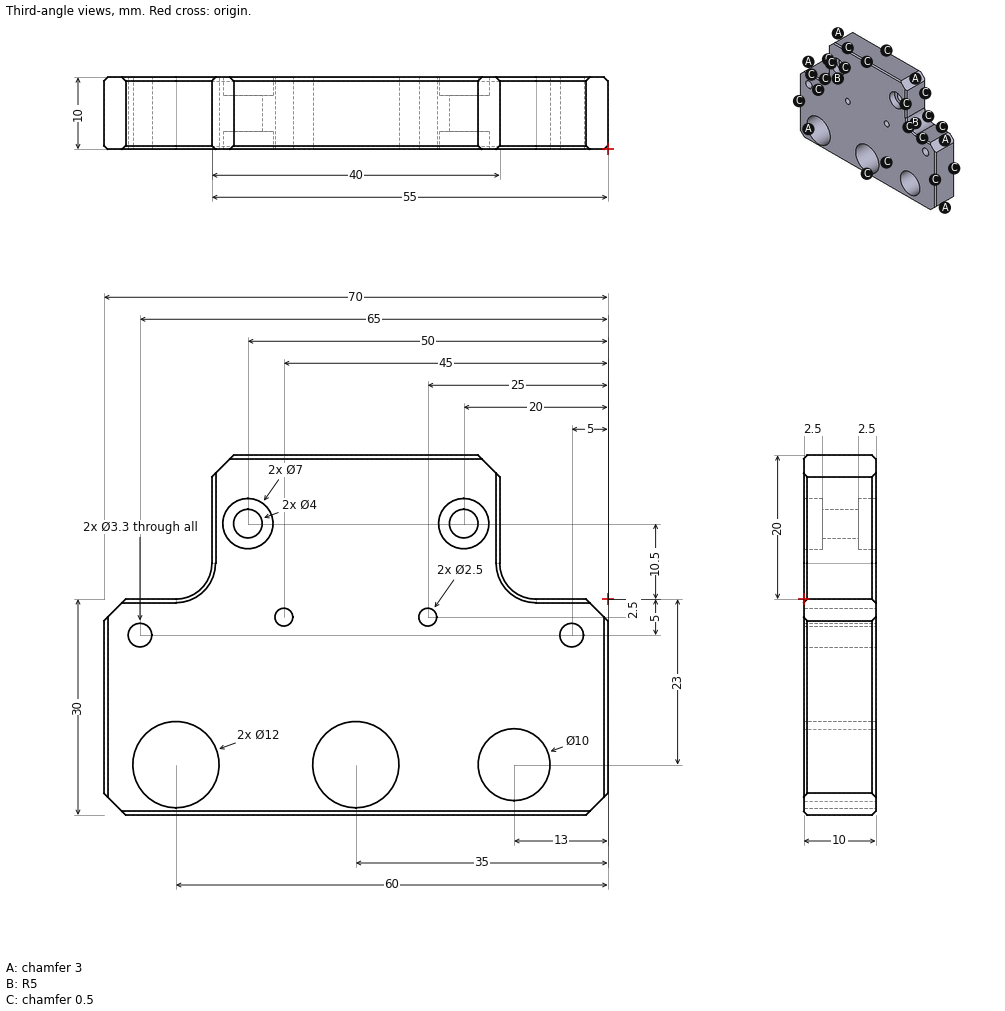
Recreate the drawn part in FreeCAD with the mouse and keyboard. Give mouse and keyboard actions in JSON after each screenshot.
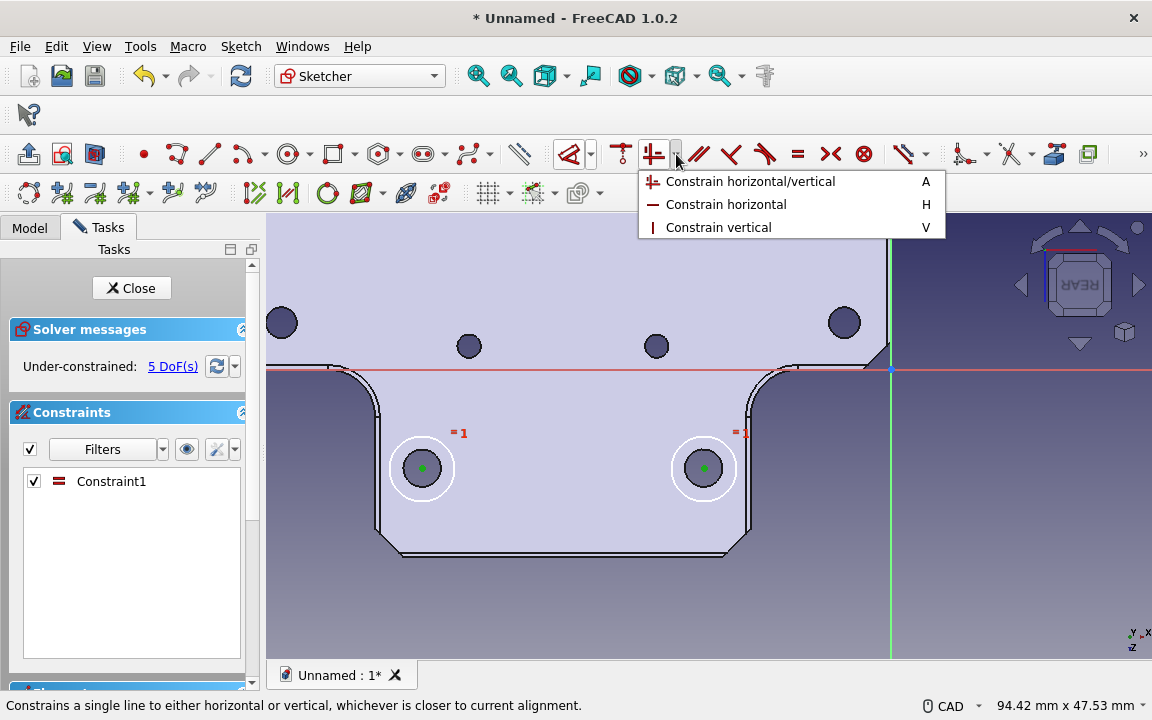
{"action": "left_click", "coordinate": [792, 204]}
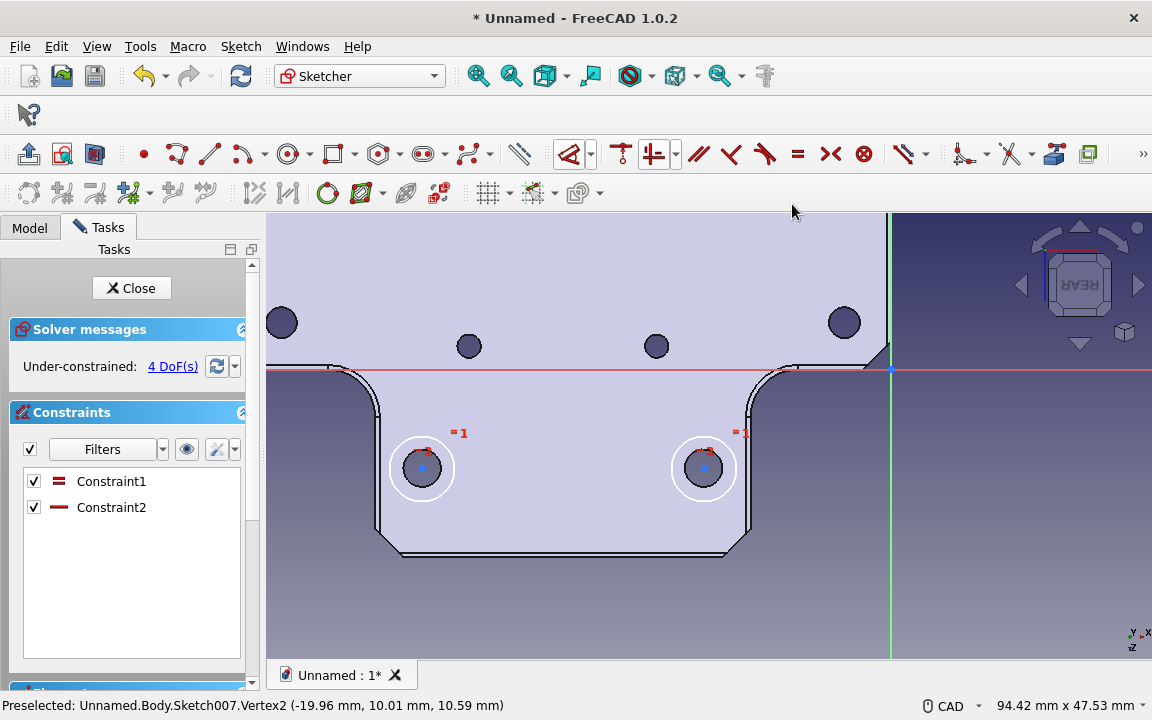
{"action": "left_click", "coordinate": [445, 446]}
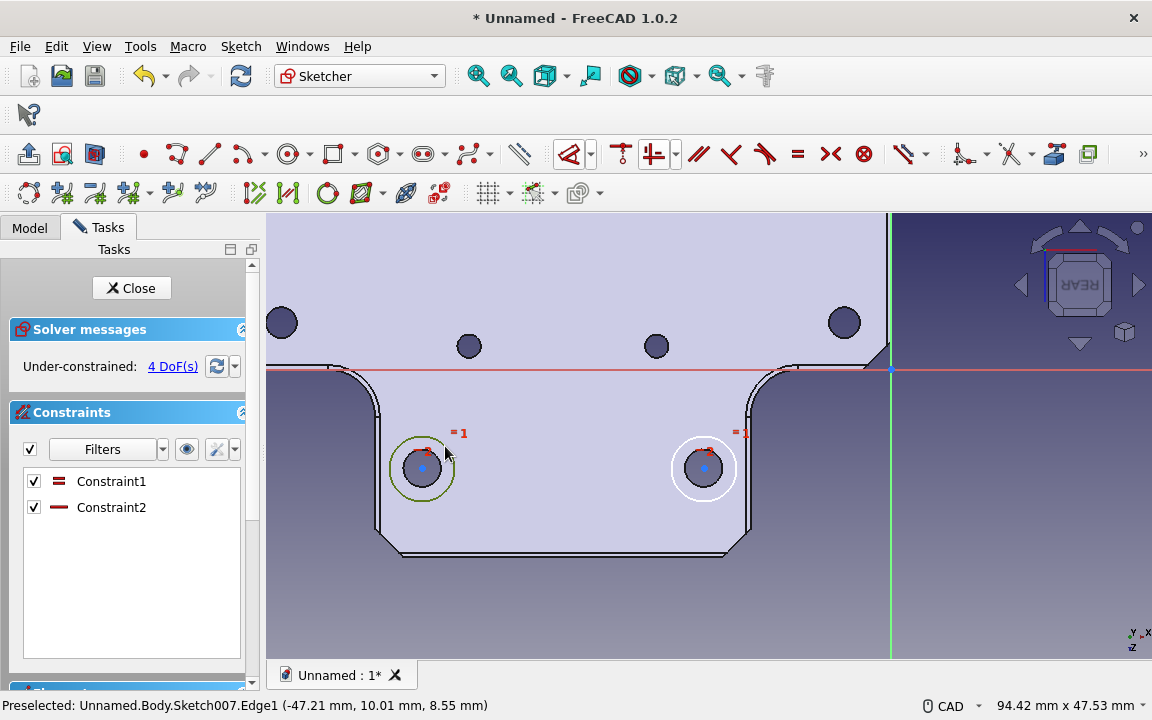
{"action": "key", "text": "k o"}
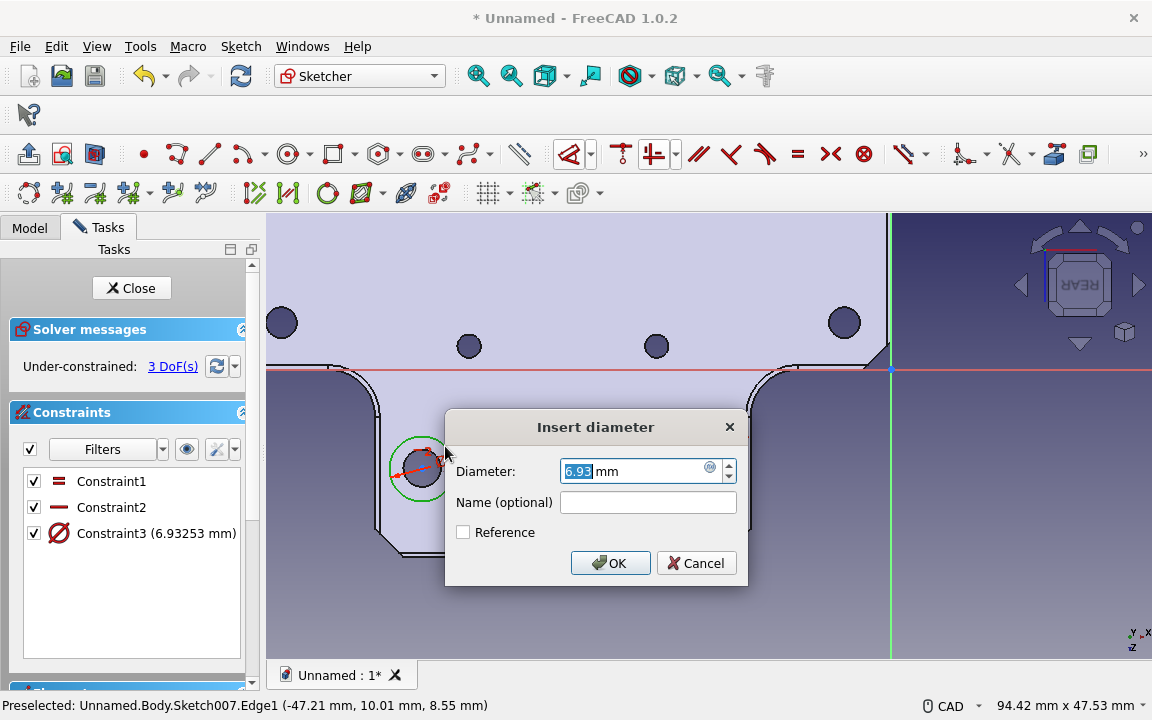
{"action": "type", "text": "7"}
{"action": "key", "text": "Return"}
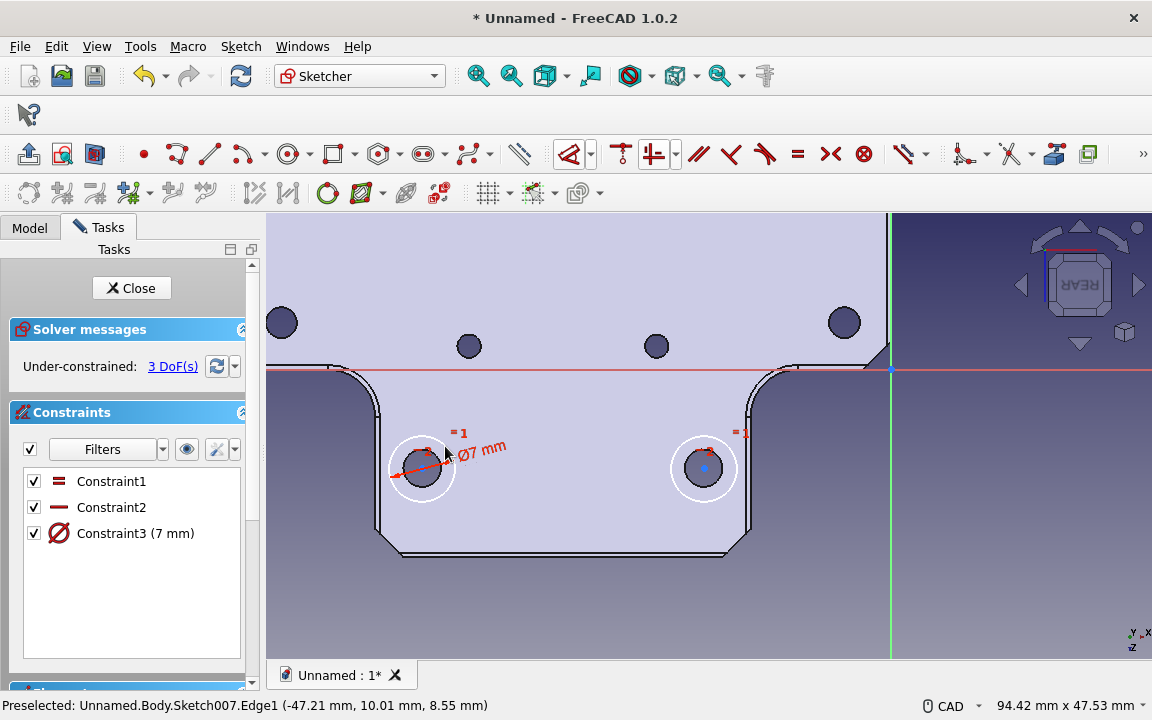
{"action": "left_click", "coordinate": [422, 469]}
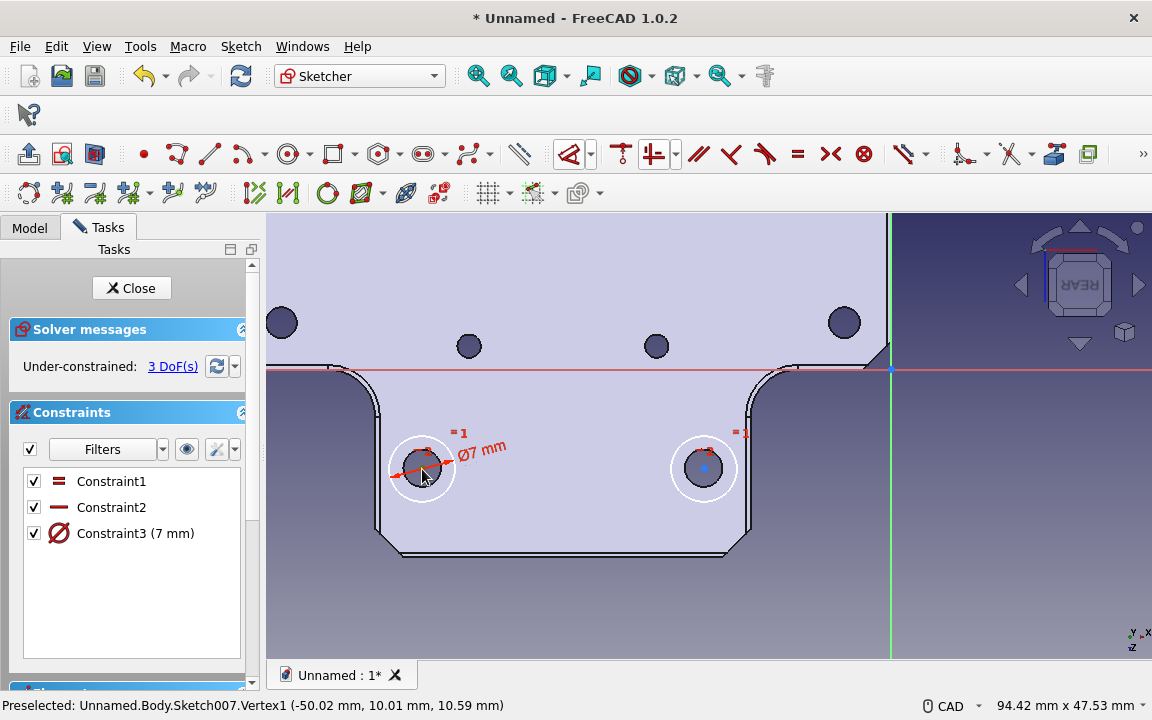
{"action": "left_click", "coordinate": [590, 154]}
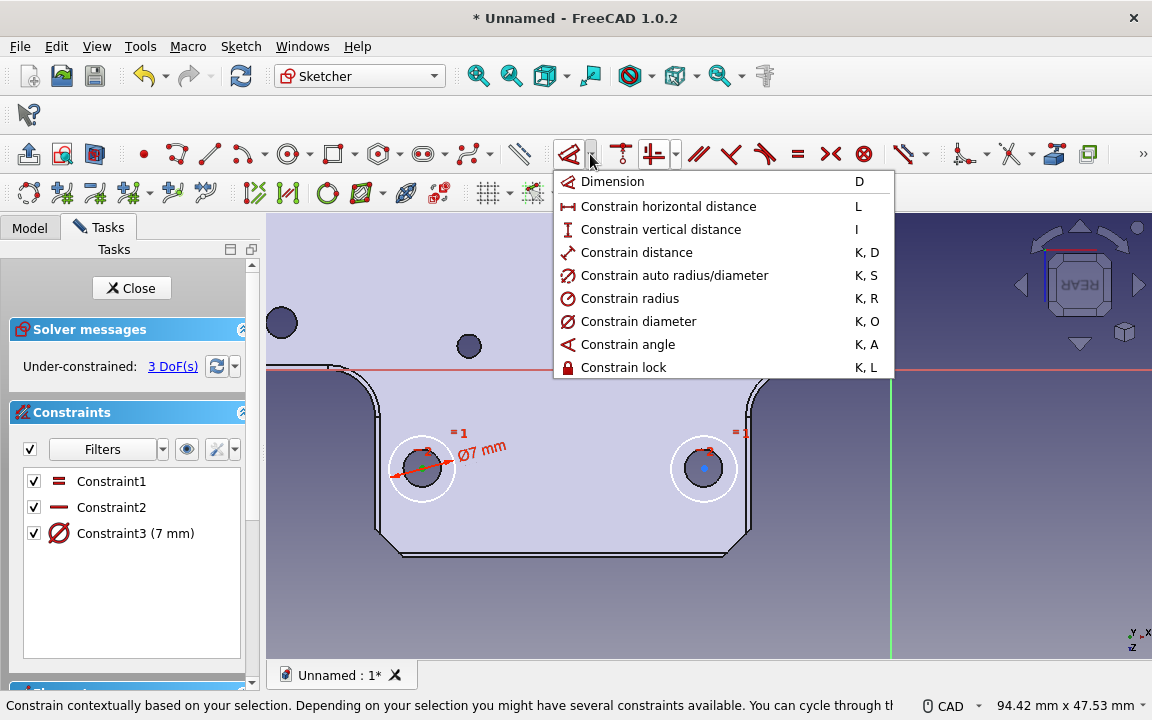
{"action": "left_click", "coordinate": [724, 206]}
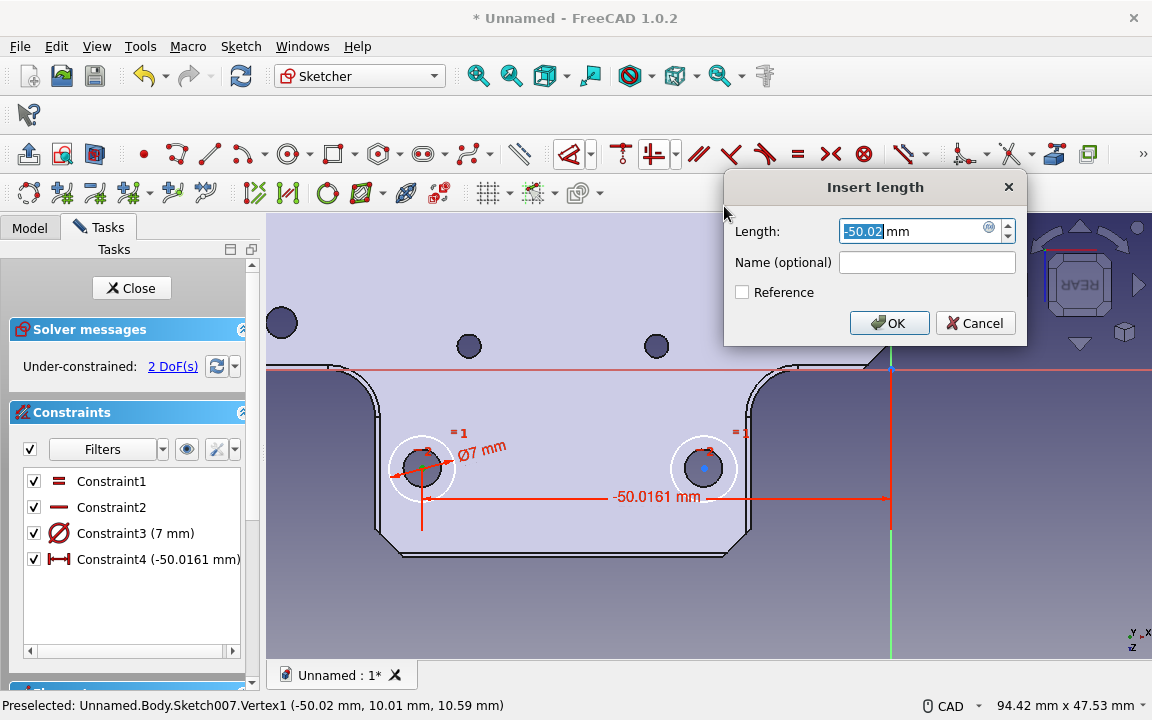
{"action": "type", "text": "-50"}
{"action": "key", "text": "Return"}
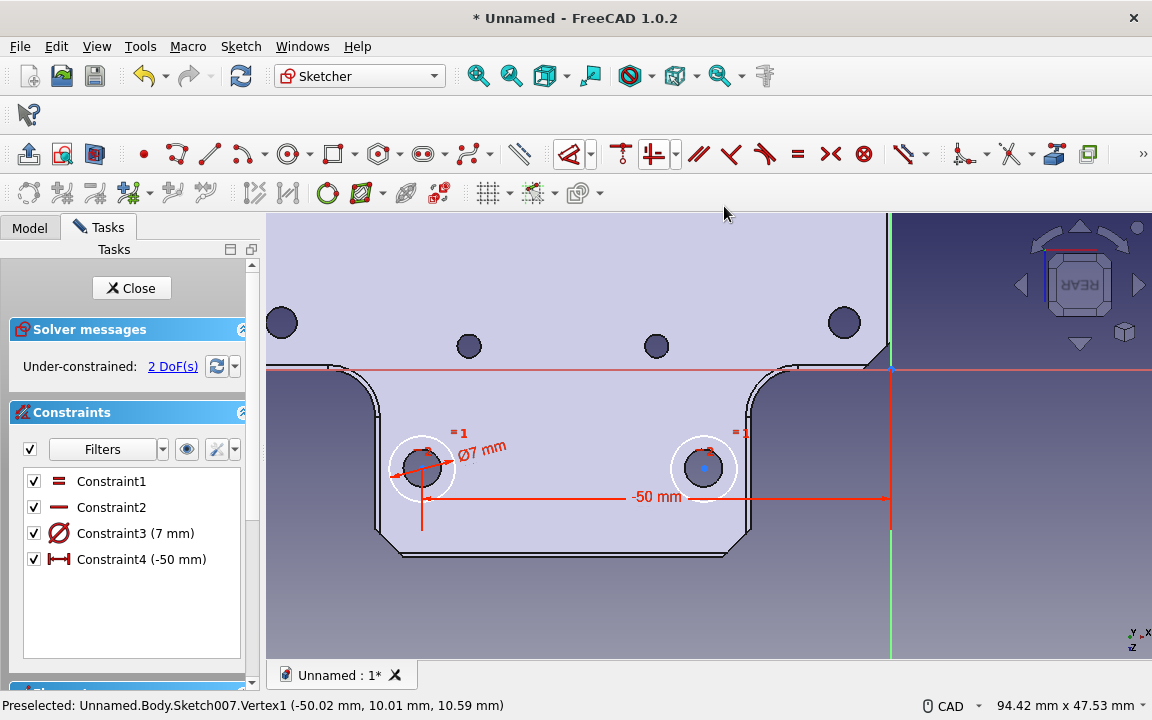
{"action": "left_click", "coordinate": [704, 469]}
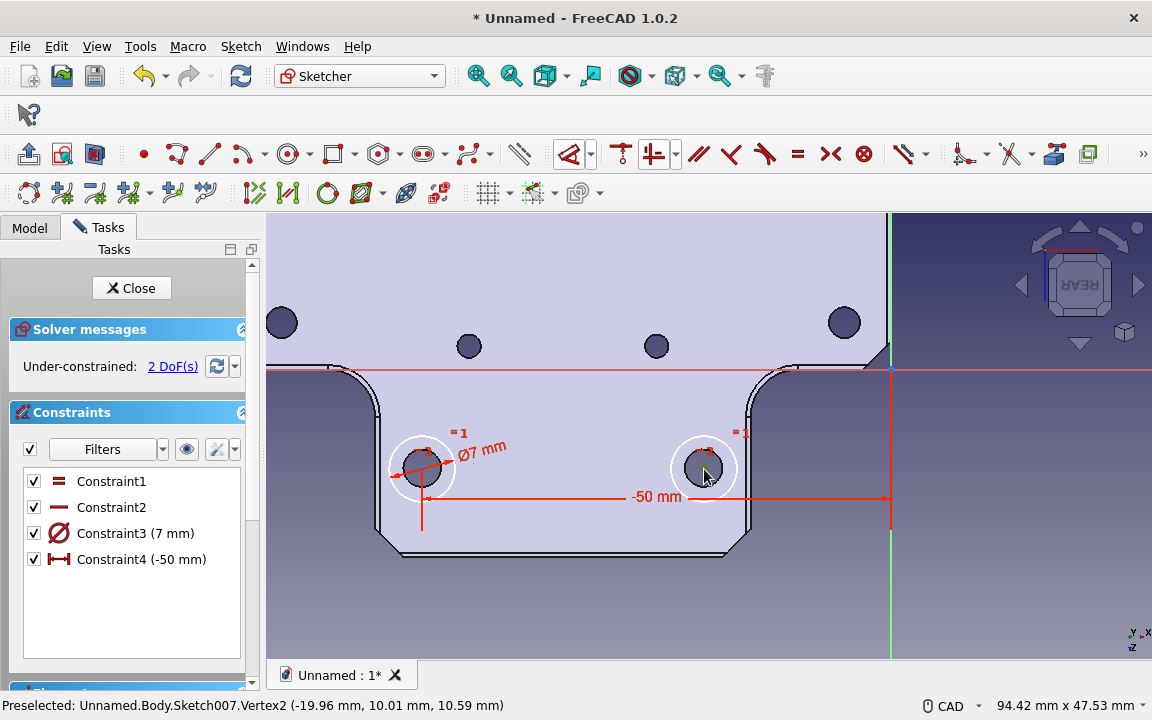
{"action": "key", "text": "l"}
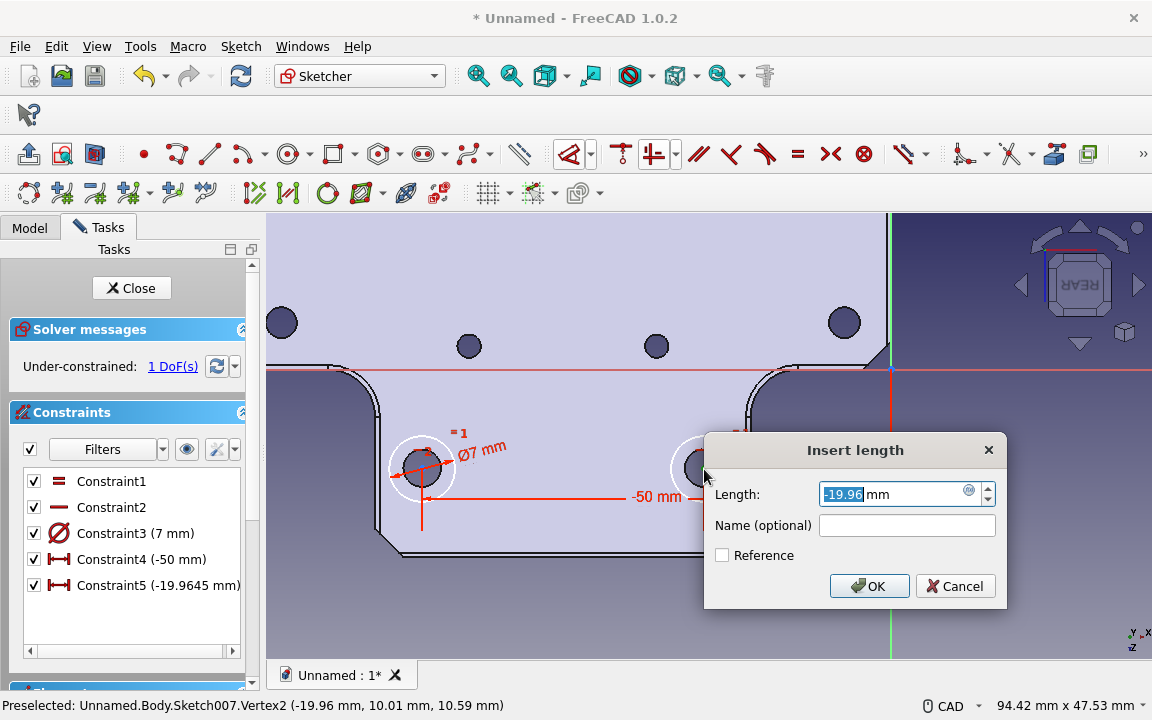
{"action": "type", "text": "-20"}
{"action": "key", "text": "Return"}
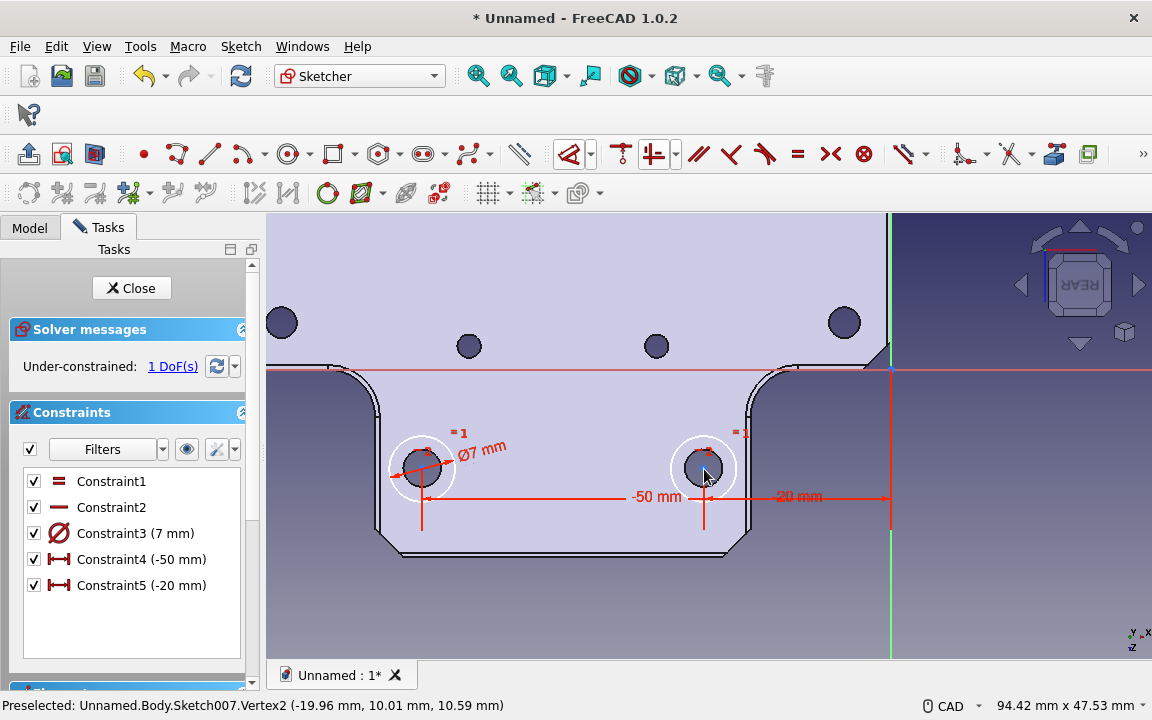
{"action": "left_click", "coordinate": [422, 469]}